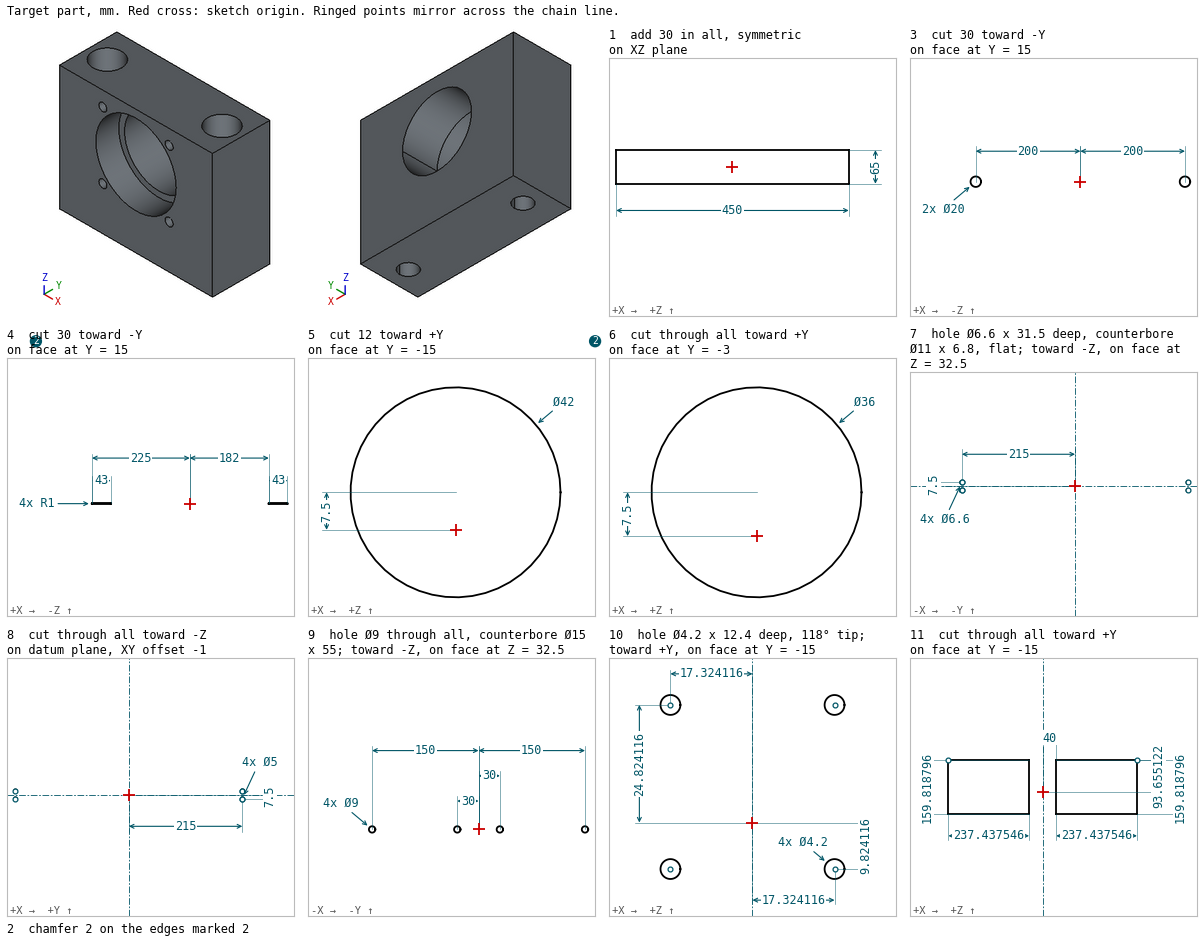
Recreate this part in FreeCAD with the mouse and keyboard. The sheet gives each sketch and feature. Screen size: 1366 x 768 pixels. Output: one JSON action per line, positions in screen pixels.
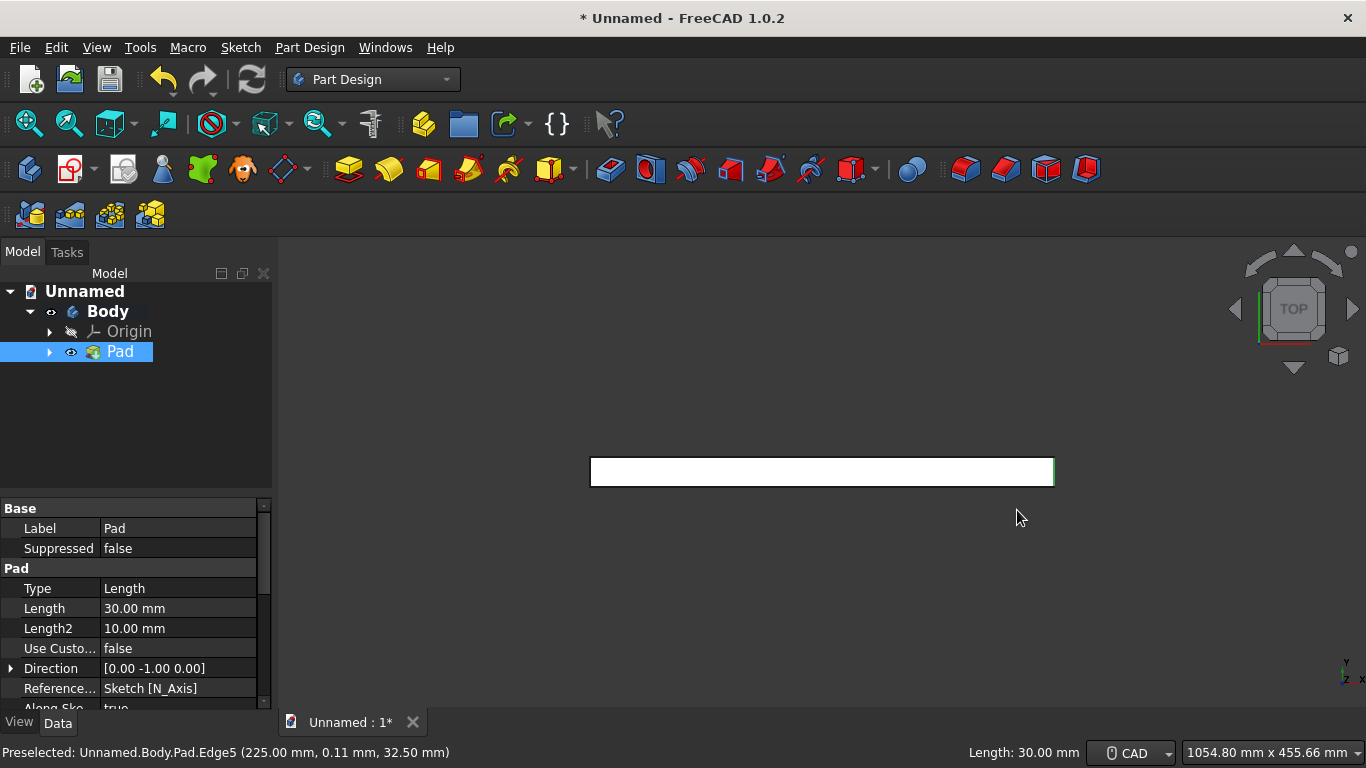
{"action": "left_click", "coordinate": [590, 471], "text": "ctrl"}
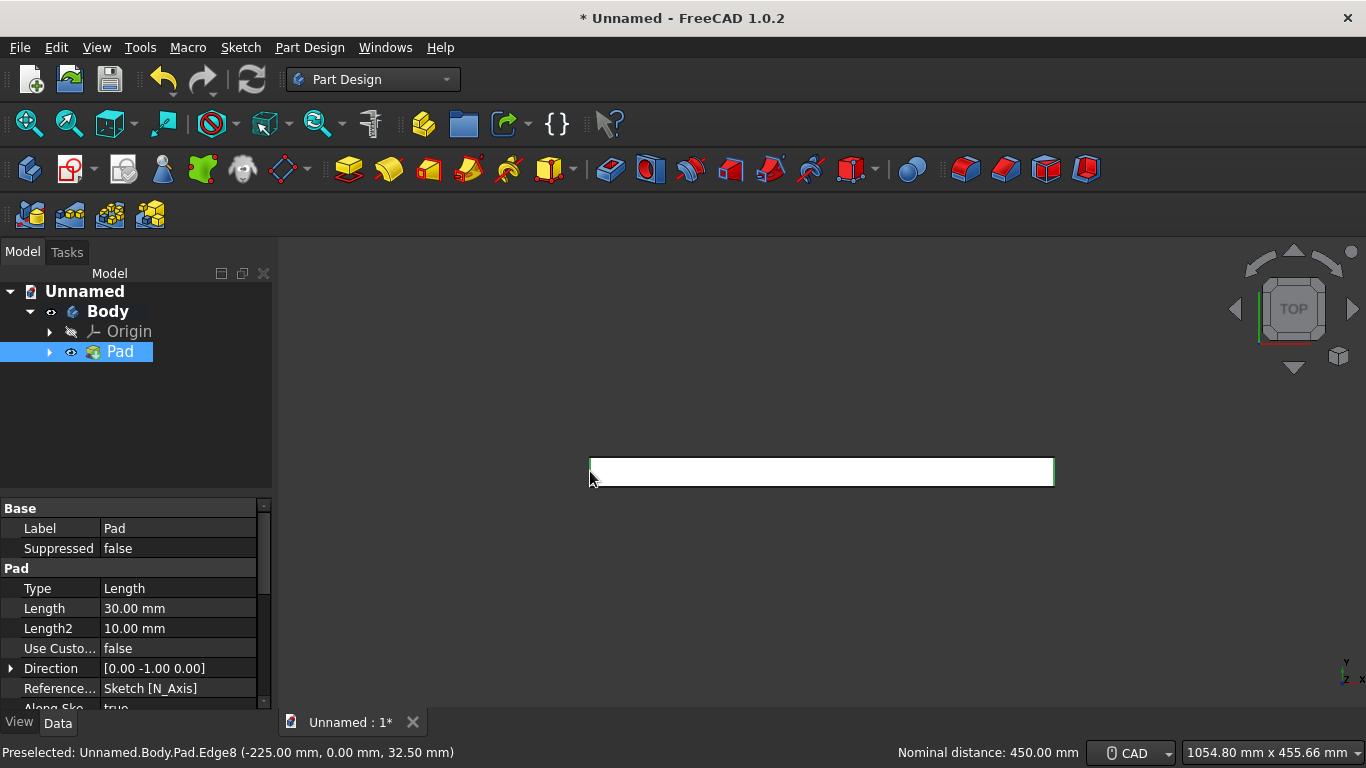
{"action": "left_click", "coordinate": [1006, 170]}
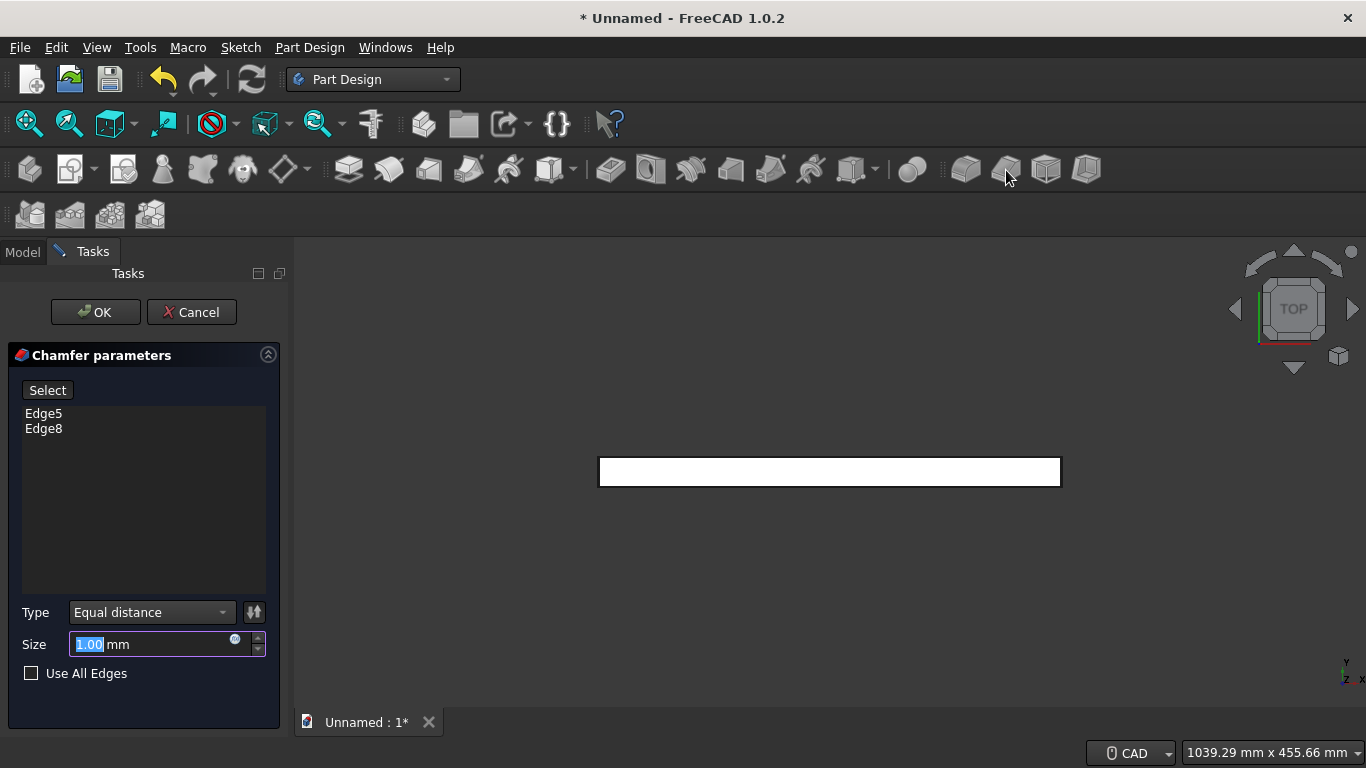
{"action": "type", "text": "2"}
{"action": "key", "text": "Tab"}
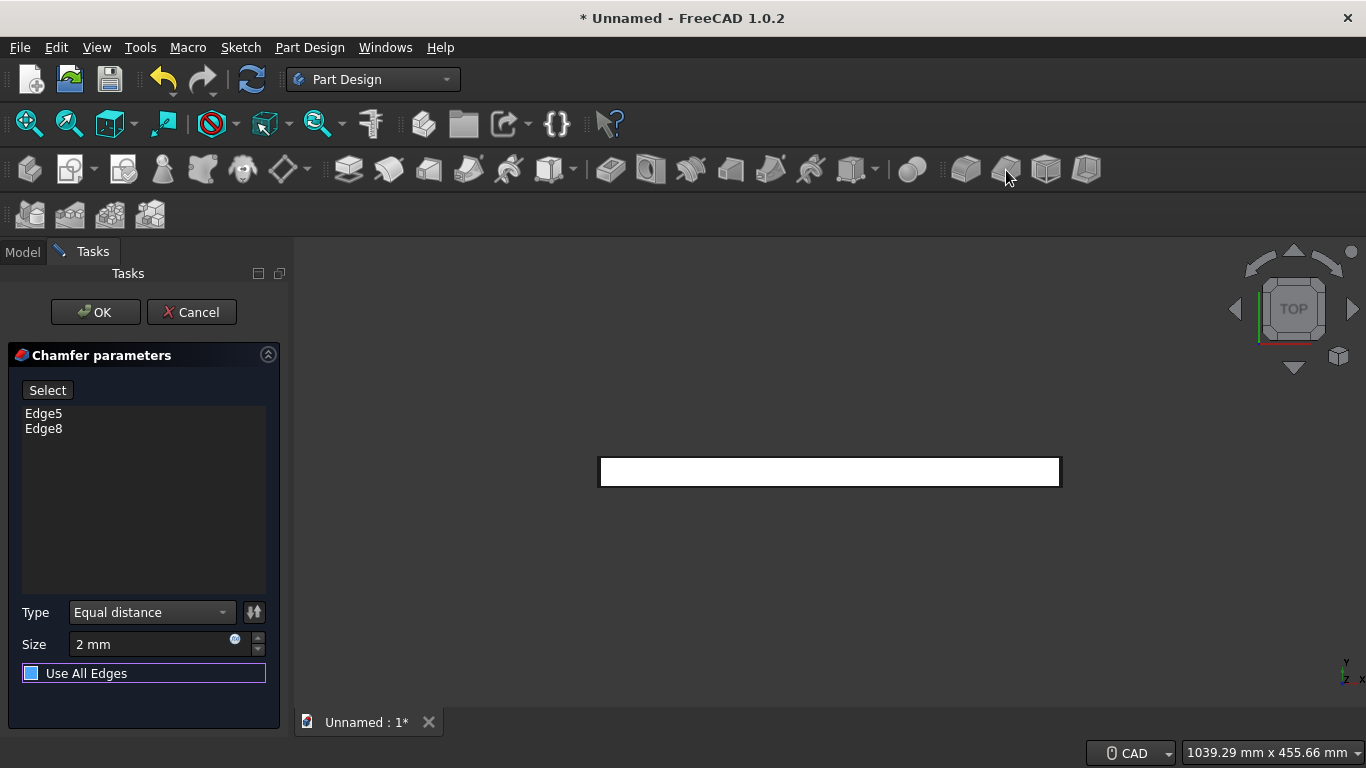
{"action": "left_click", "coordinate": [96, 312]}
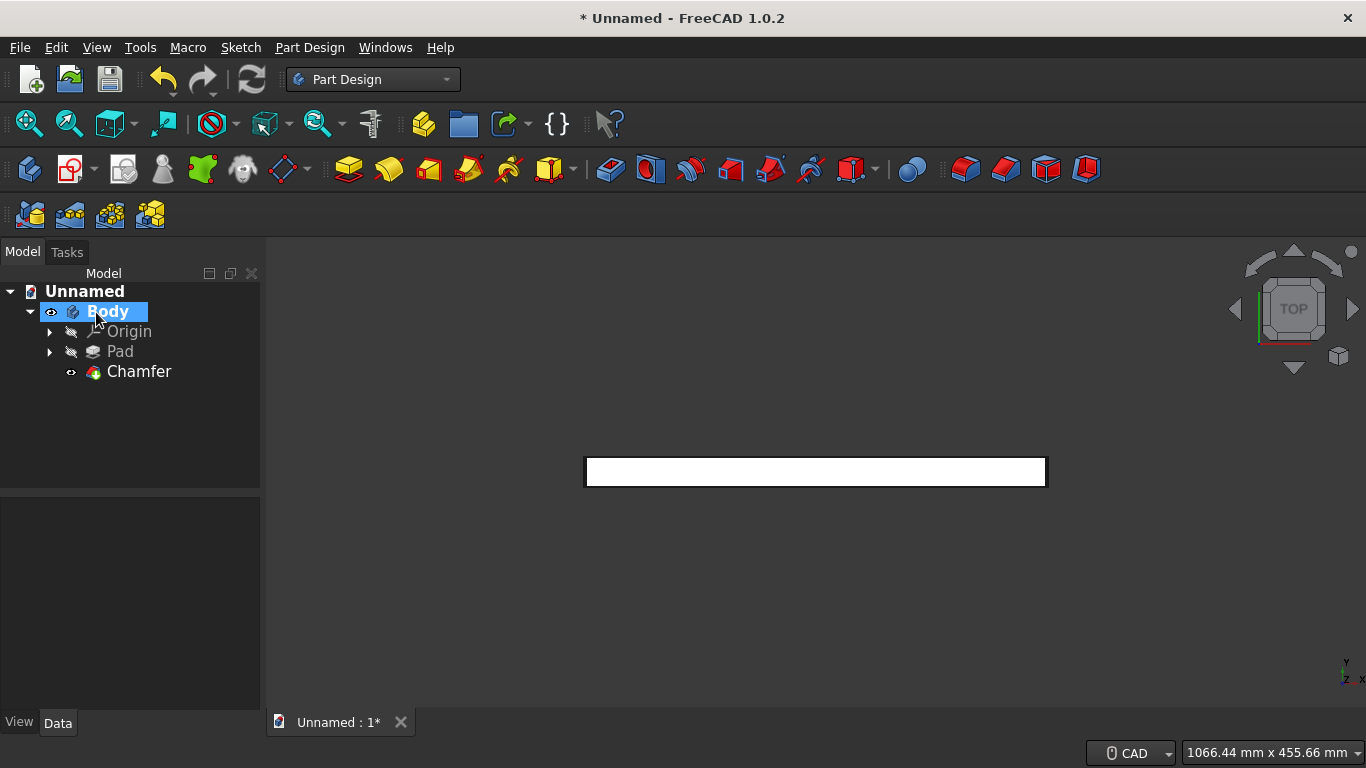
{"action": "left_click", "coordinate": [30, 124]}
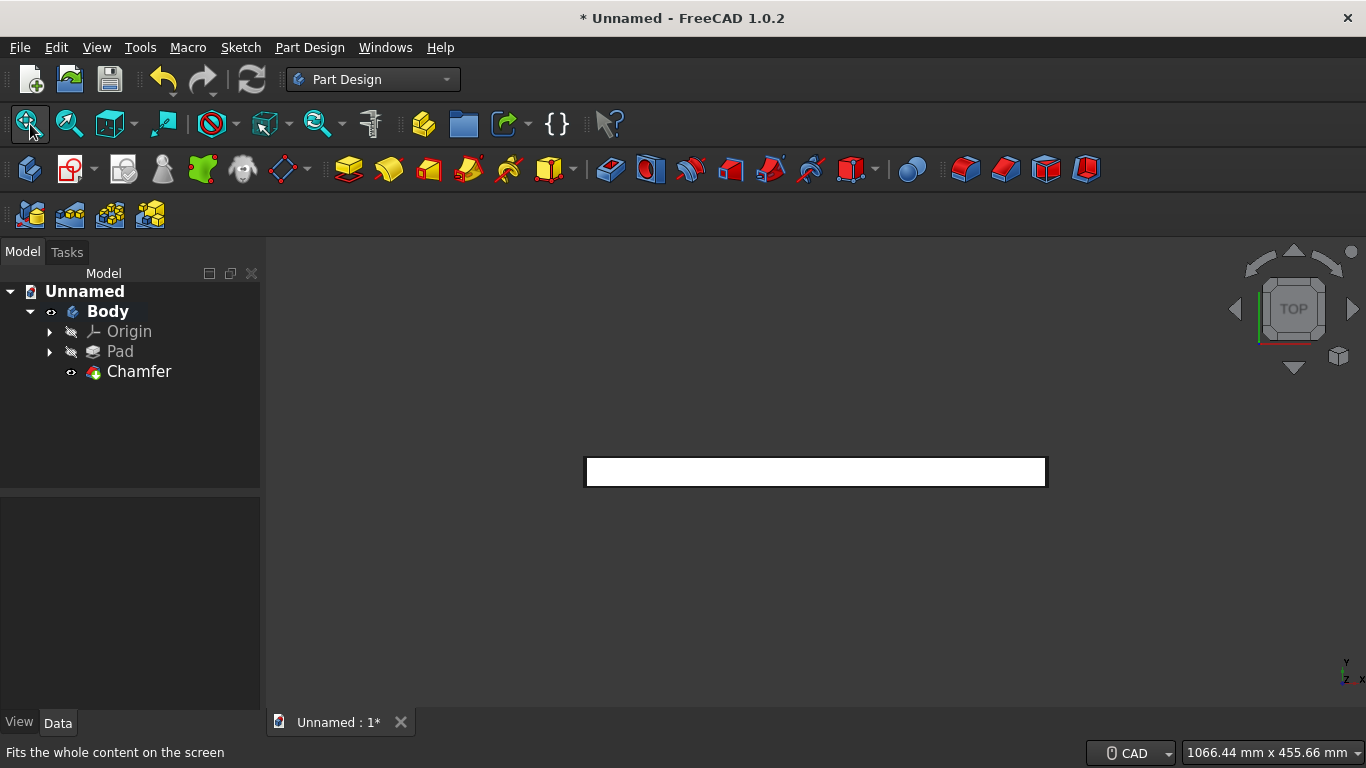
{"action": "key", "text": "4"}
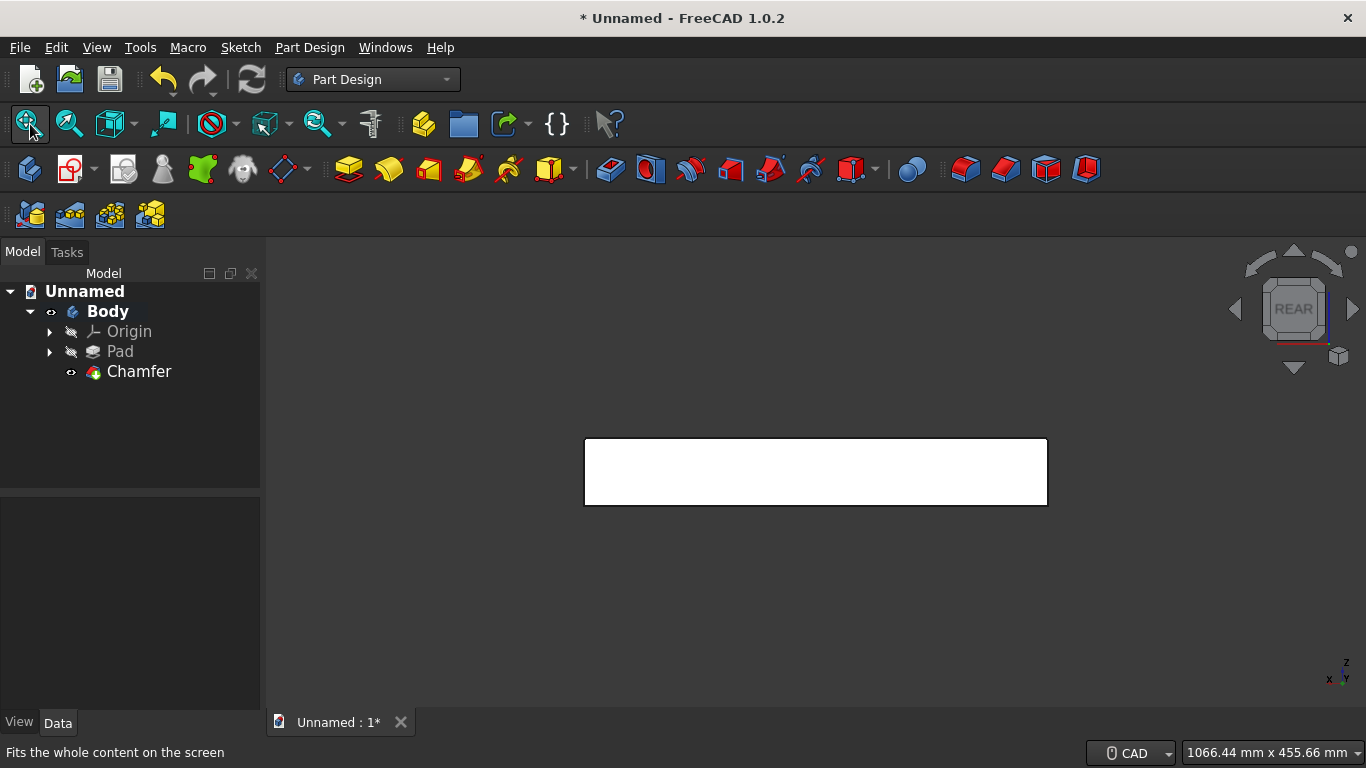
{"action": "key", "text": "v f"}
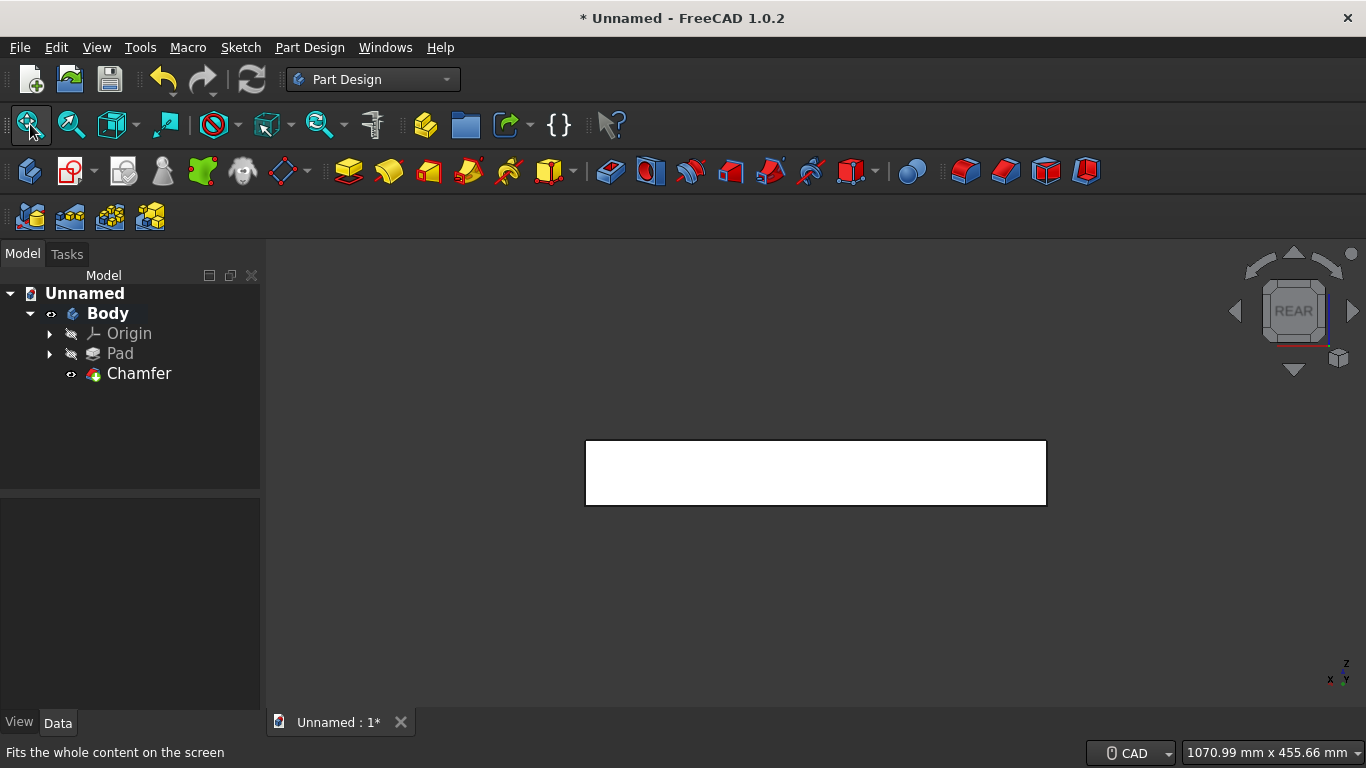
{"action": "left_click", "coordinate": [684, 472]}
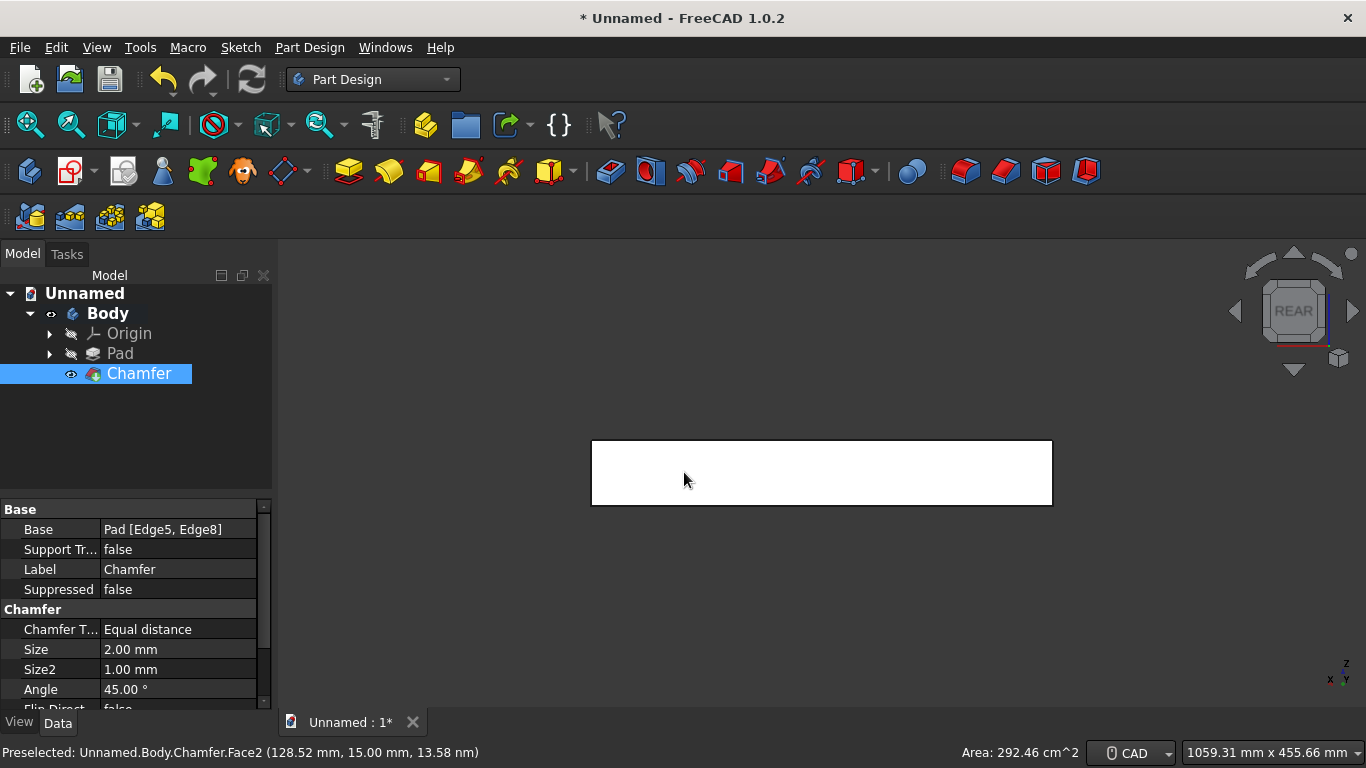
{"action": "left_click", "coordinate": [70, 172]}